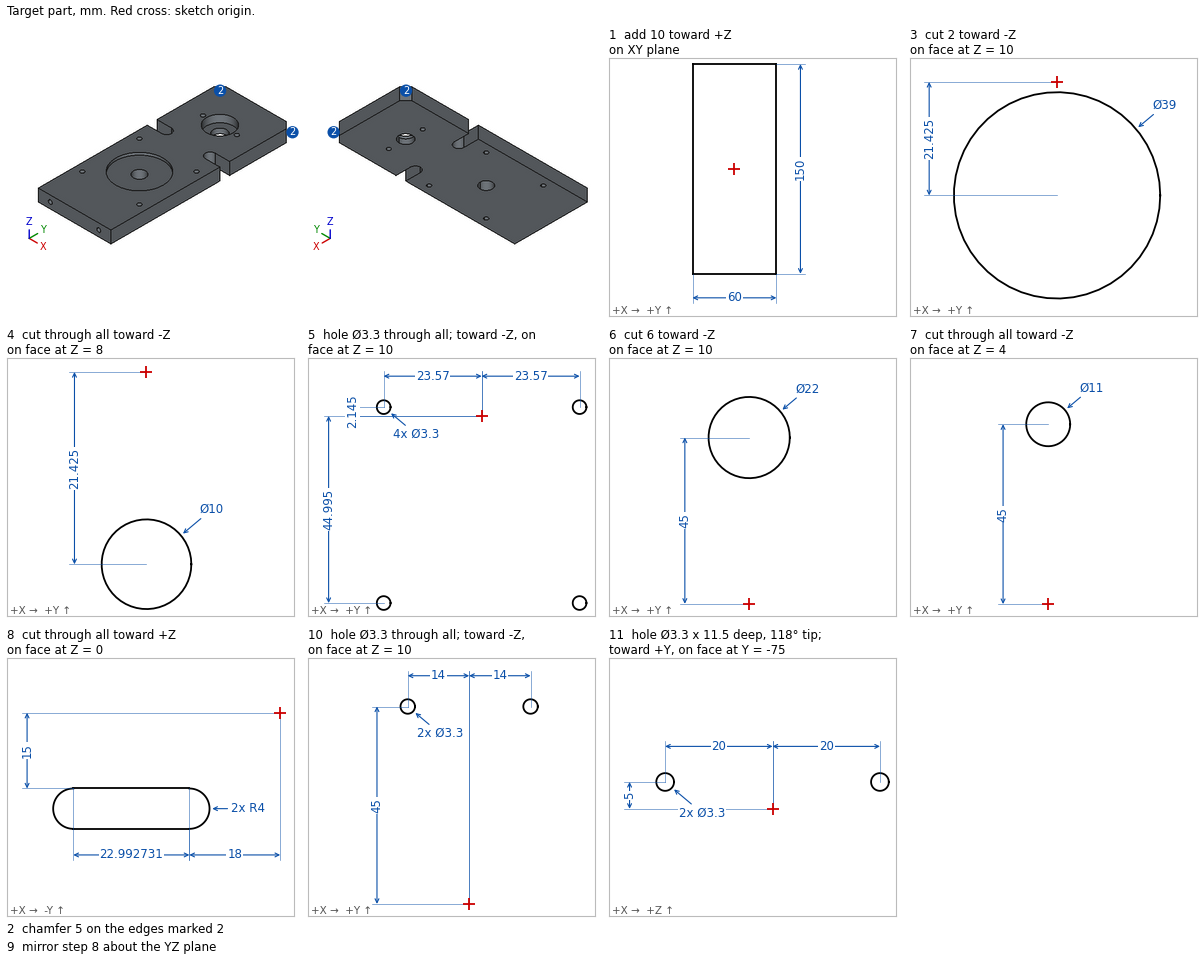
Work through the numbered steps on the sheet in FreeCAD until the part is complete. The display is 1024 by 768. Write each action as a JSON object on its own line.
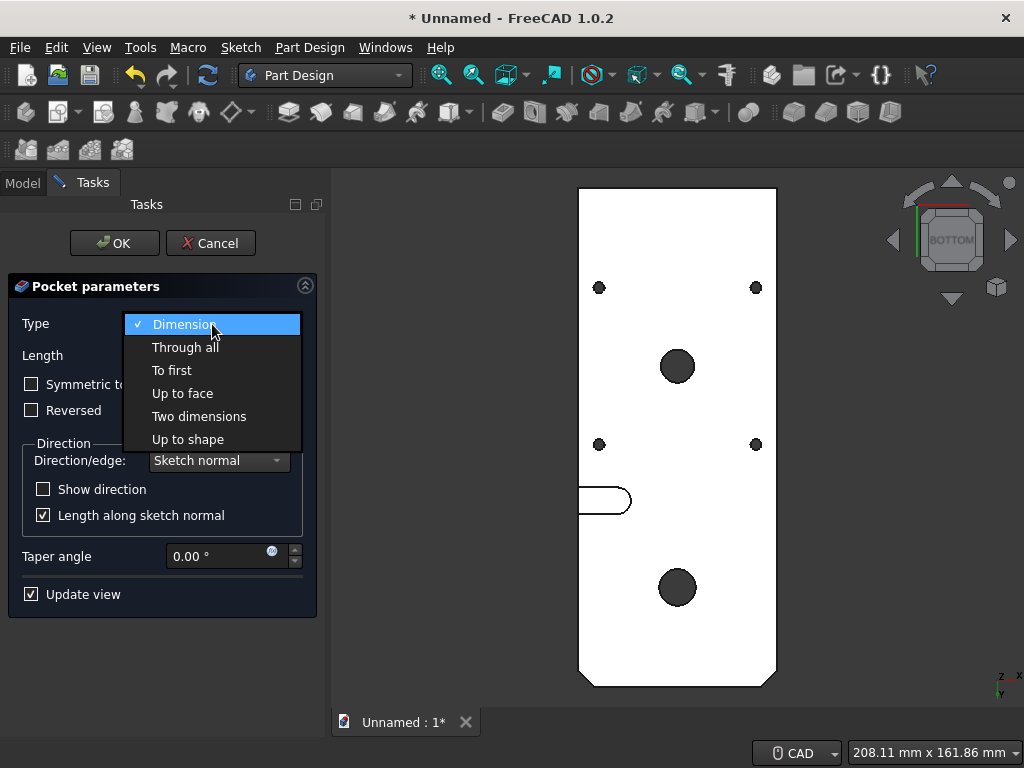
{"action": "left_click", "coordinate": [212, 348]}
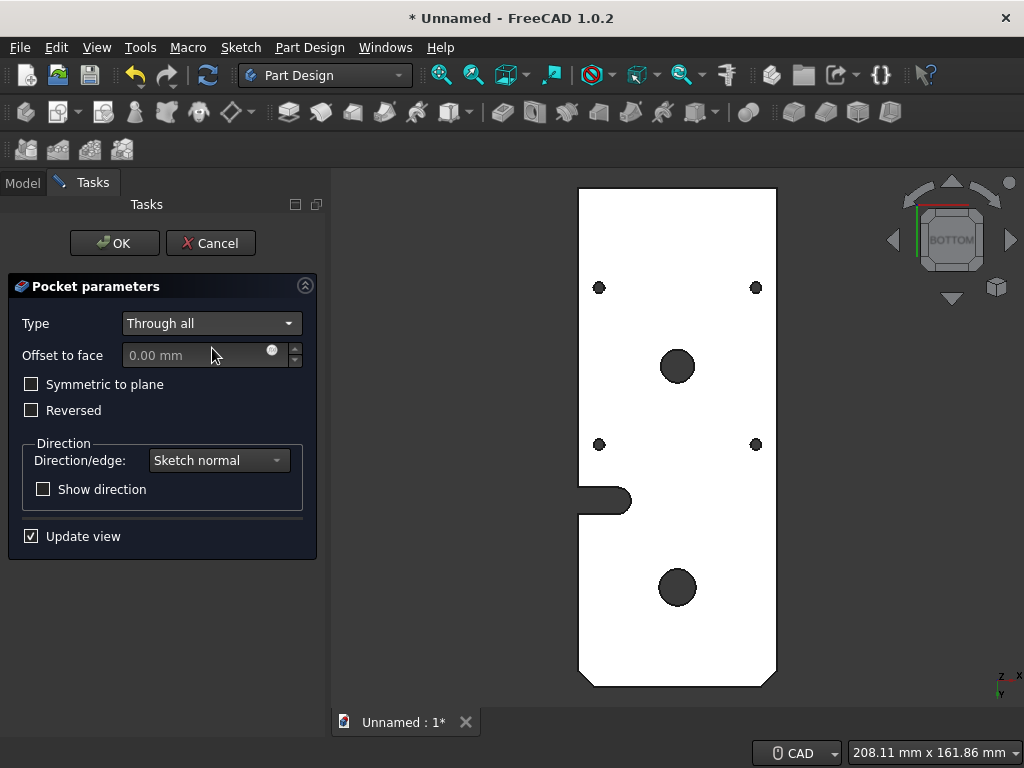
{"action": "left_click", "coordinate": [115, 243]}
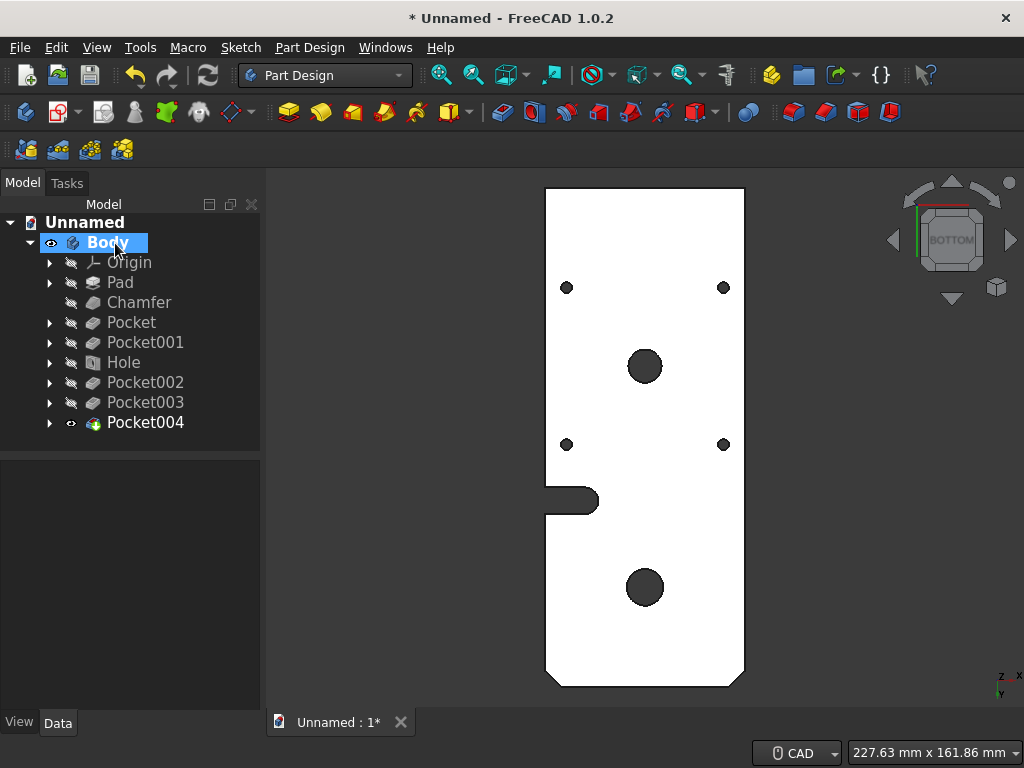
{"action": "left_click", "coordinate": [116, 423]}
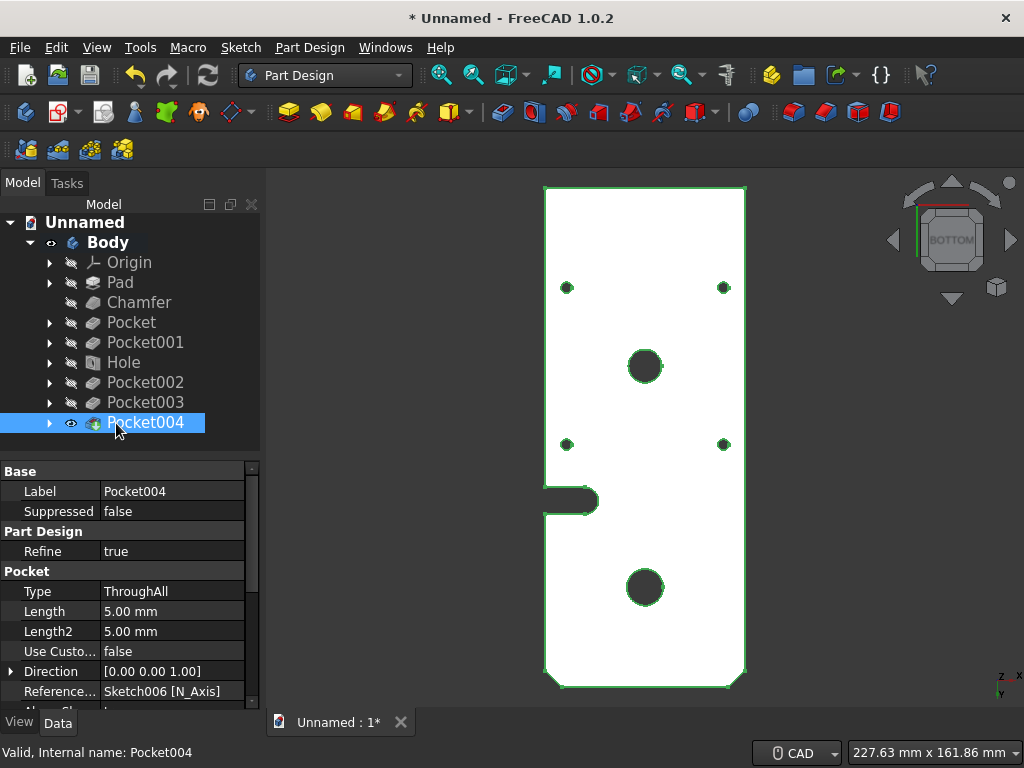
{"action": "left_click", "coordinate": [26, 150]}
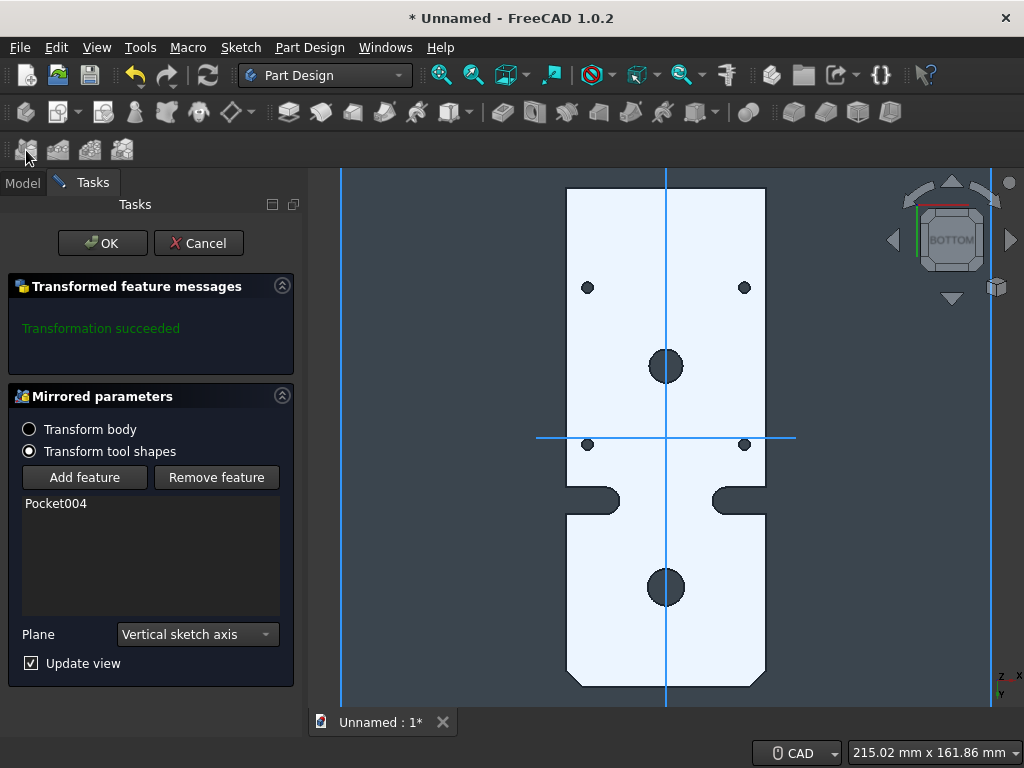
{"action": "left_click", "coordinate": [198, 634]}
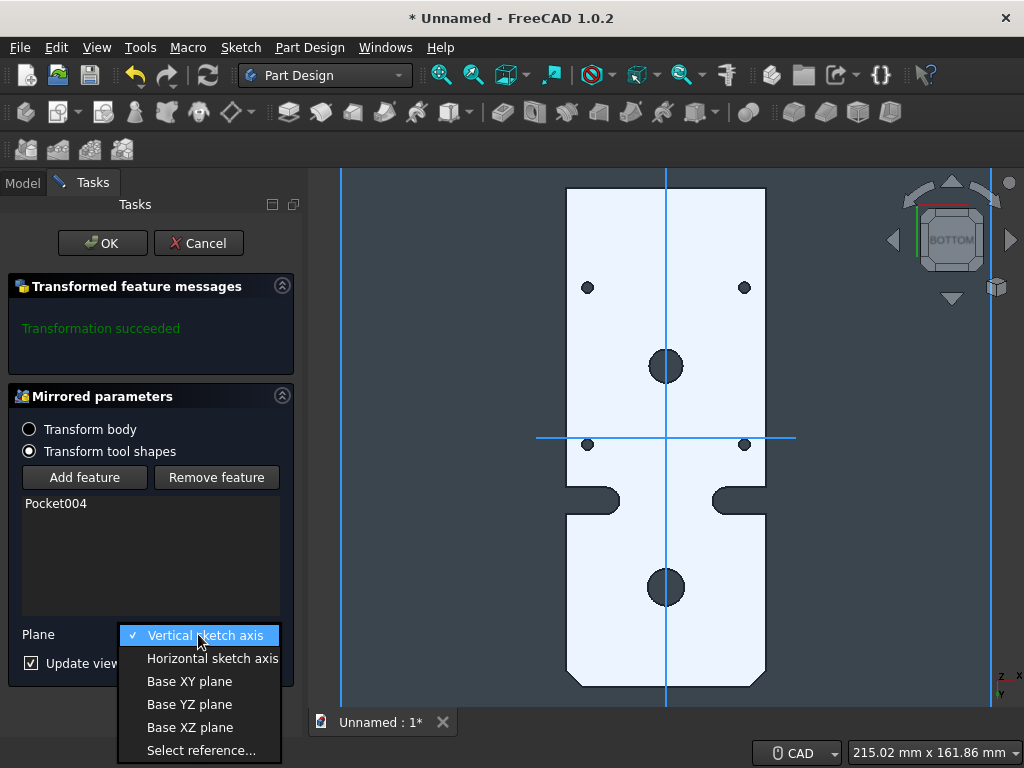
{"action": "left_click", "coordinate": [198, 704]}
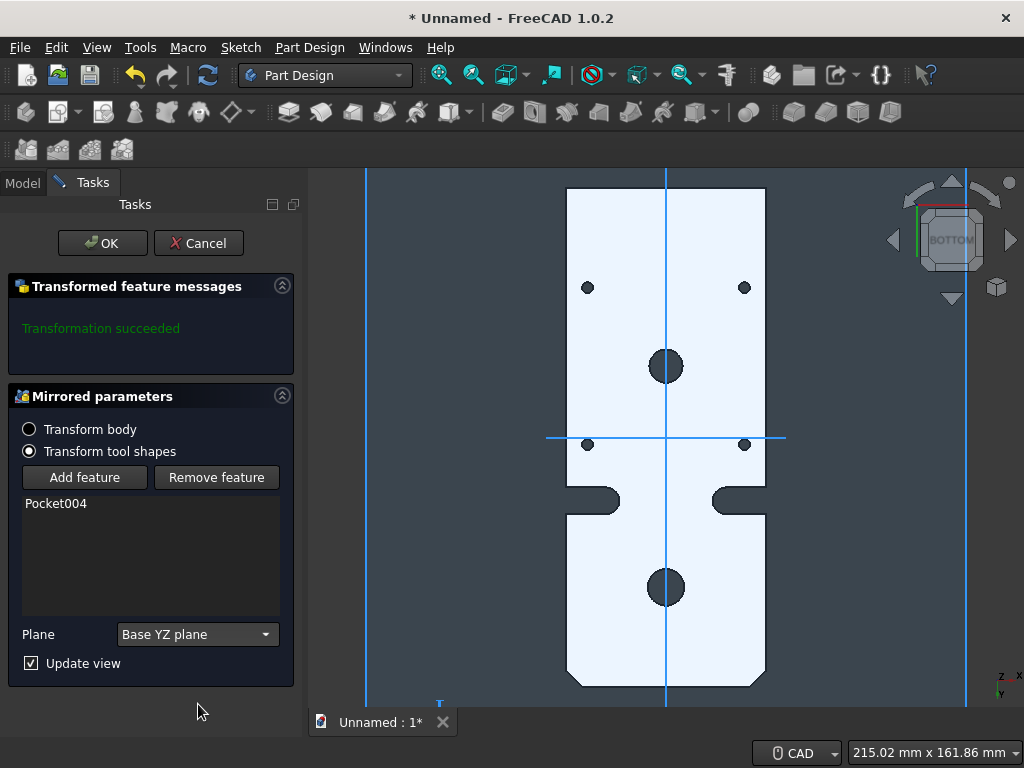
{"action": "left_click", "coordinate": [103, 243]}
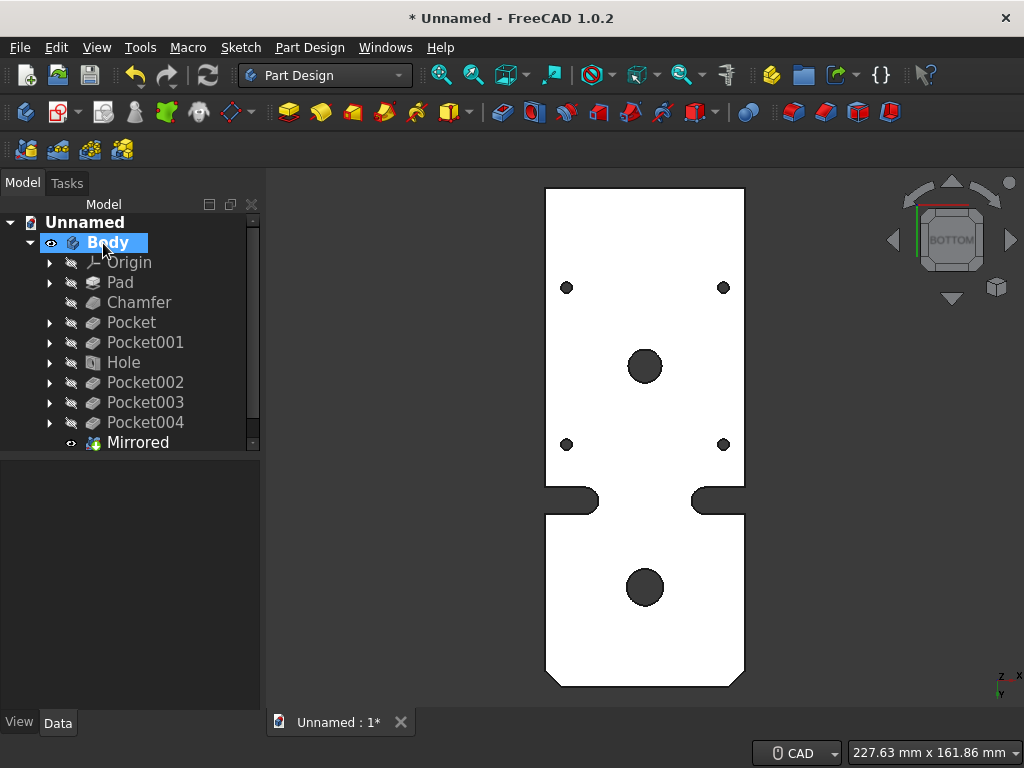
{"action": "key", "text": "0"}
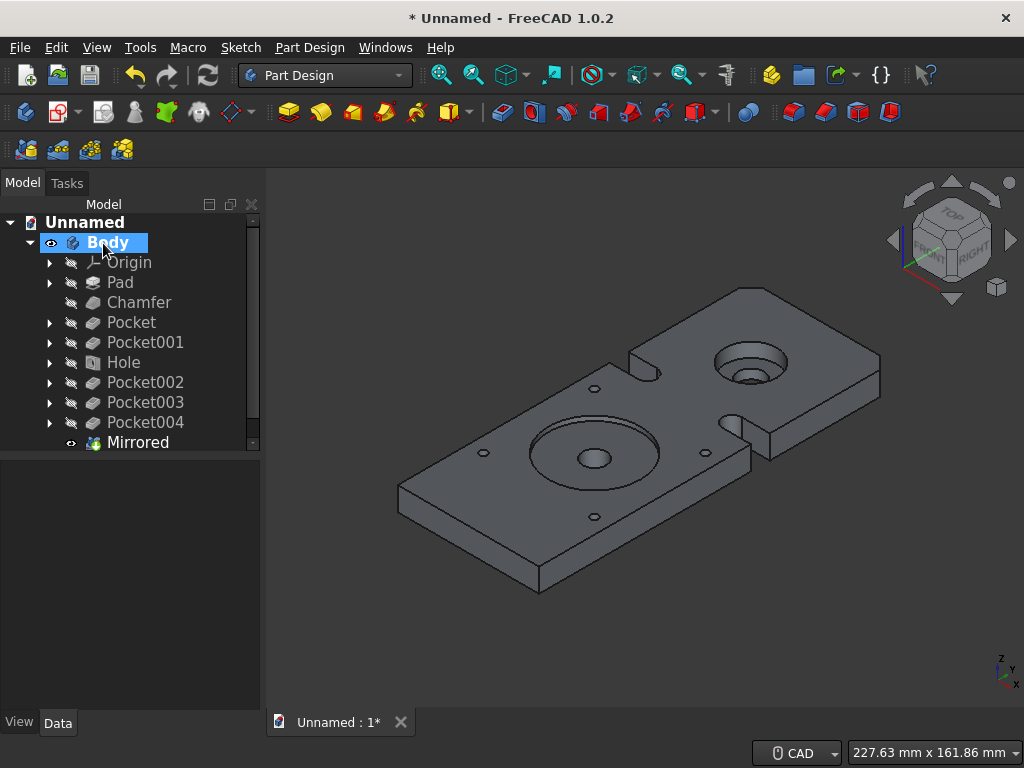
{"action": "left_click", "coordinate": [695, 394]}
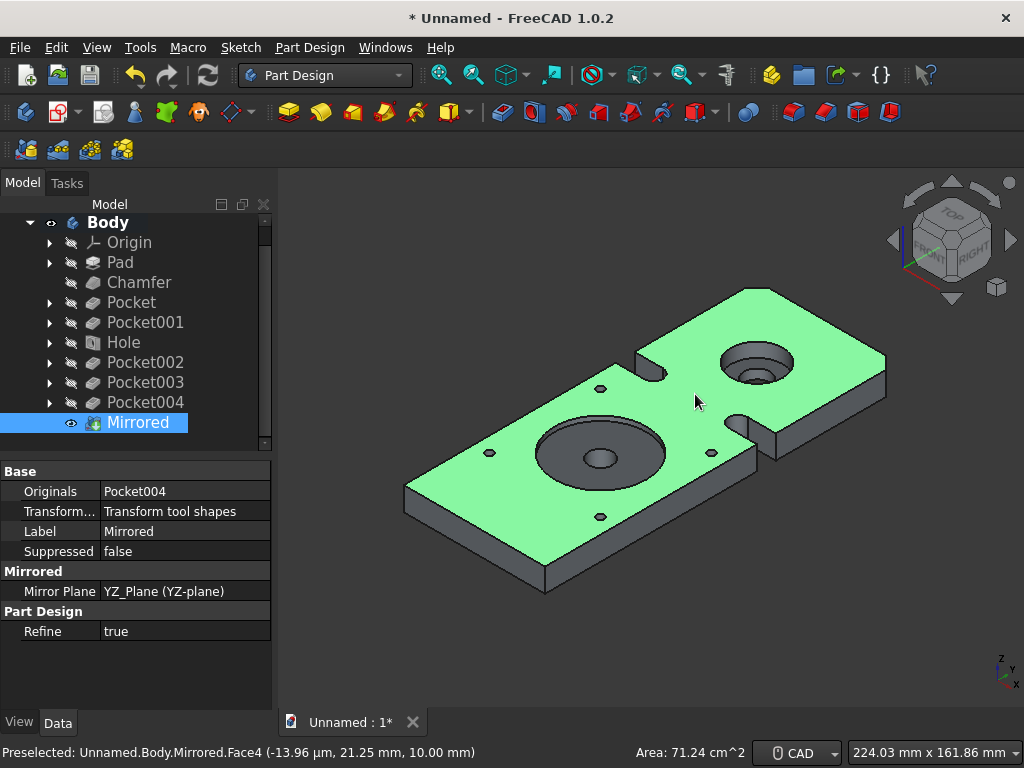
{"action": "left_click", "coordinate": [58, 112]}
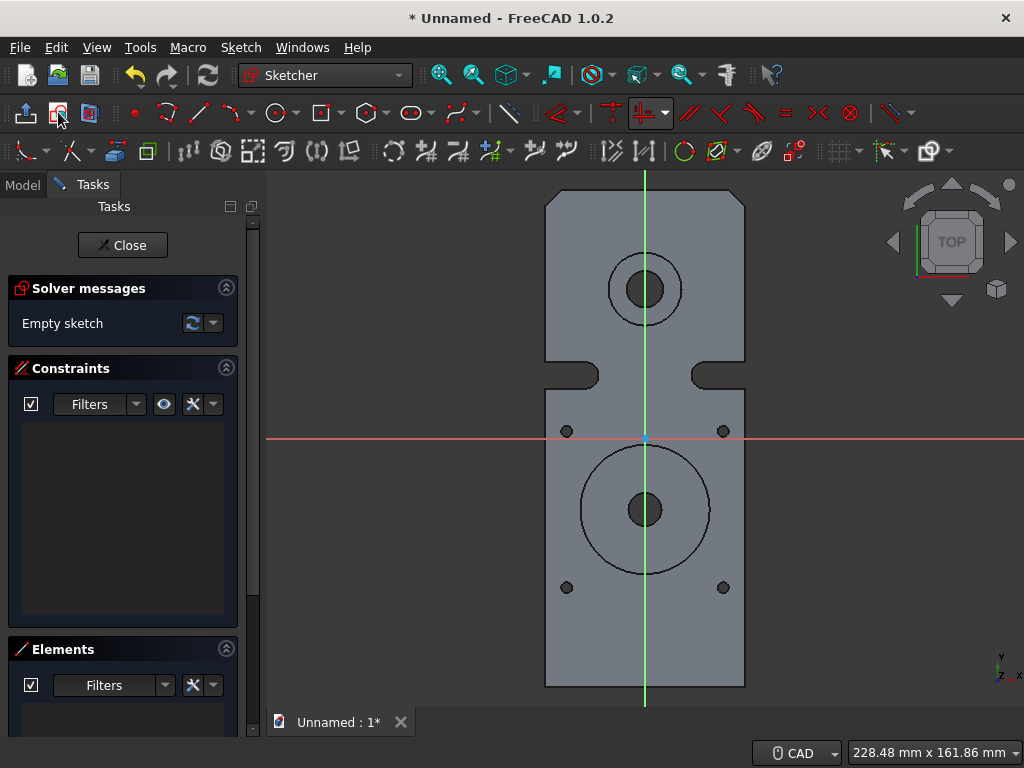
{"action": "scroll", "coordinate": [701, 298], "scroll_direction": "up", "scroll_amount": 4}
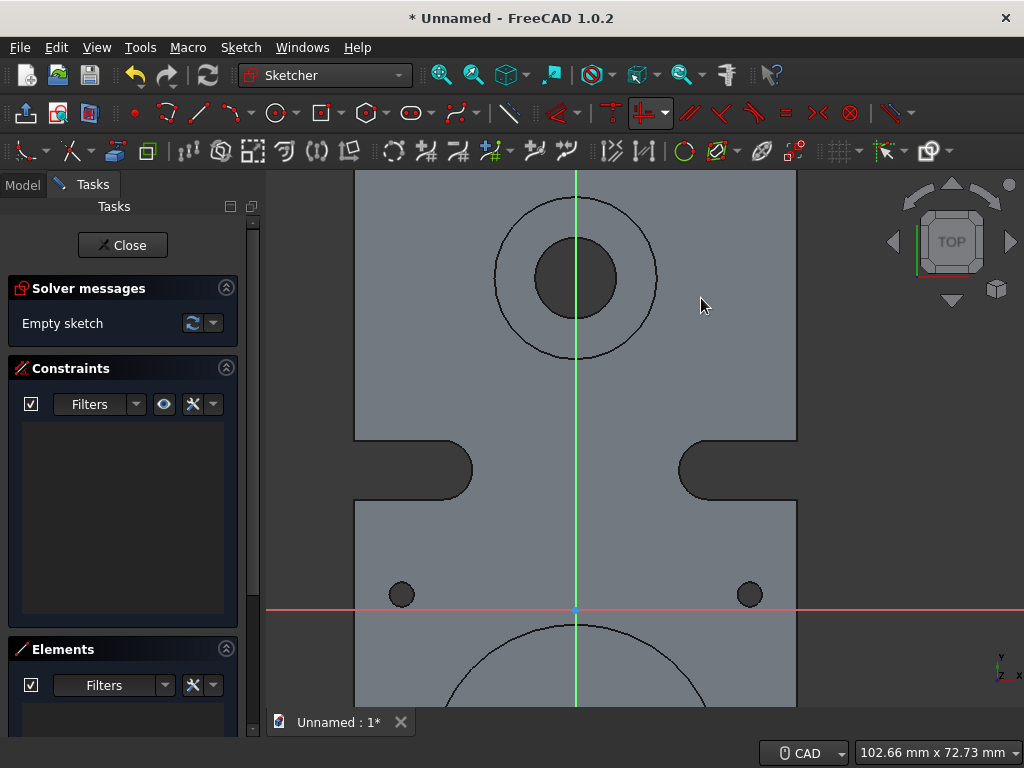
{"action": "left_click", "coordinate": [276, 114]}